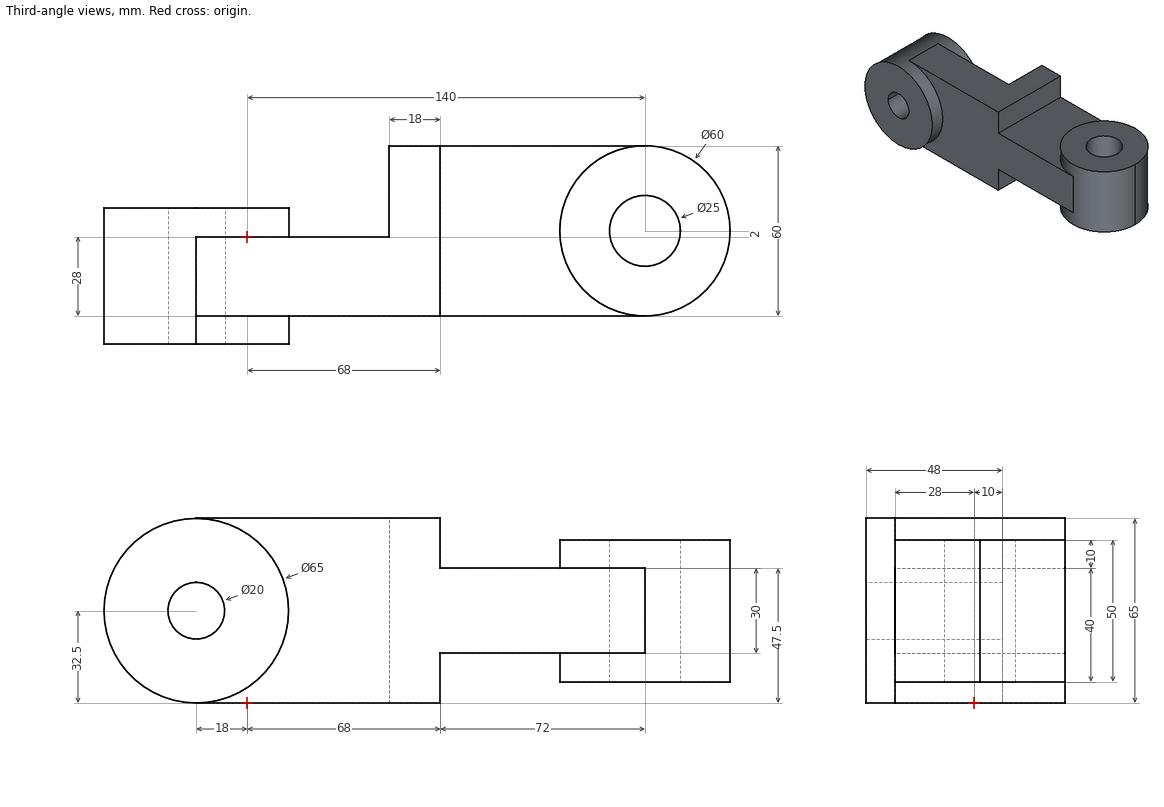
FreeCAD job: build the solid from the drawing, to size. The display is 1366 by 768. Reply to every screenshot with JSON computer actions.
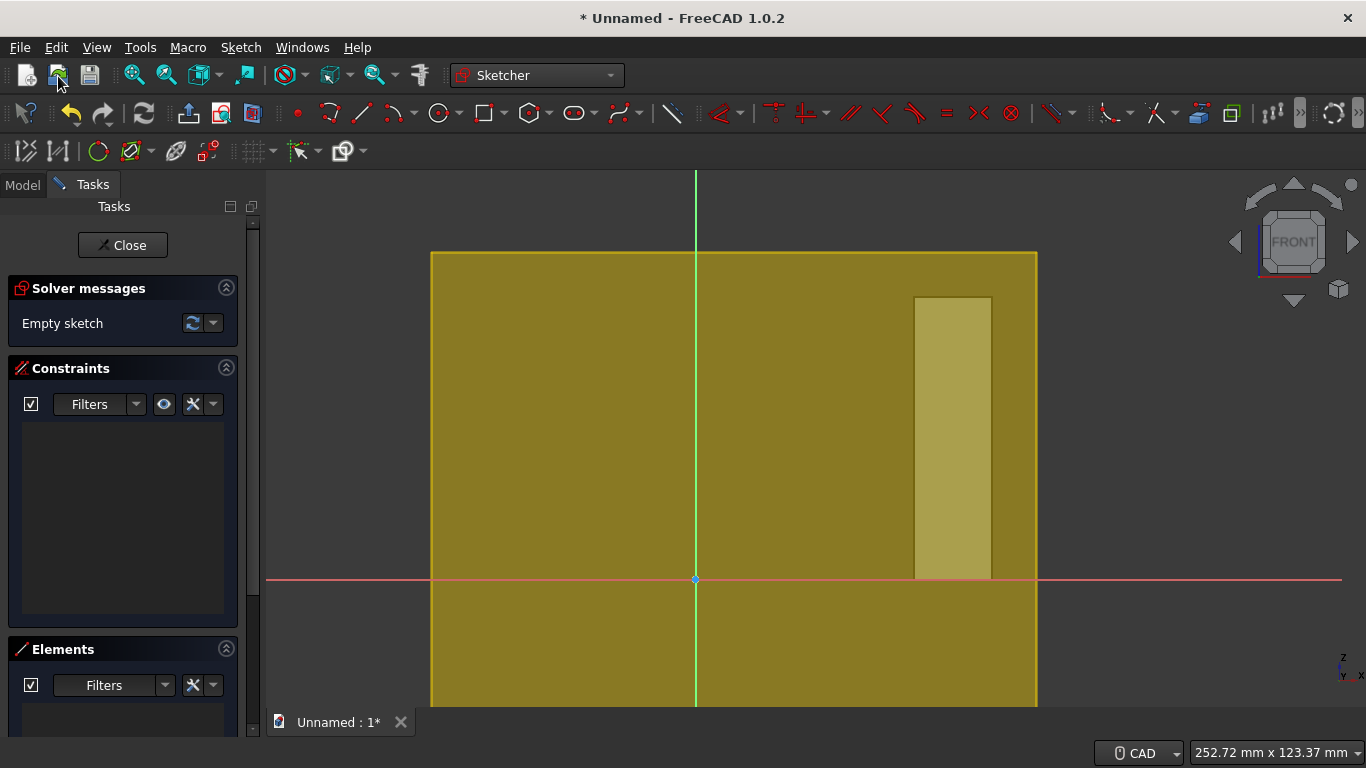
{"action": "key", "text": "g c"}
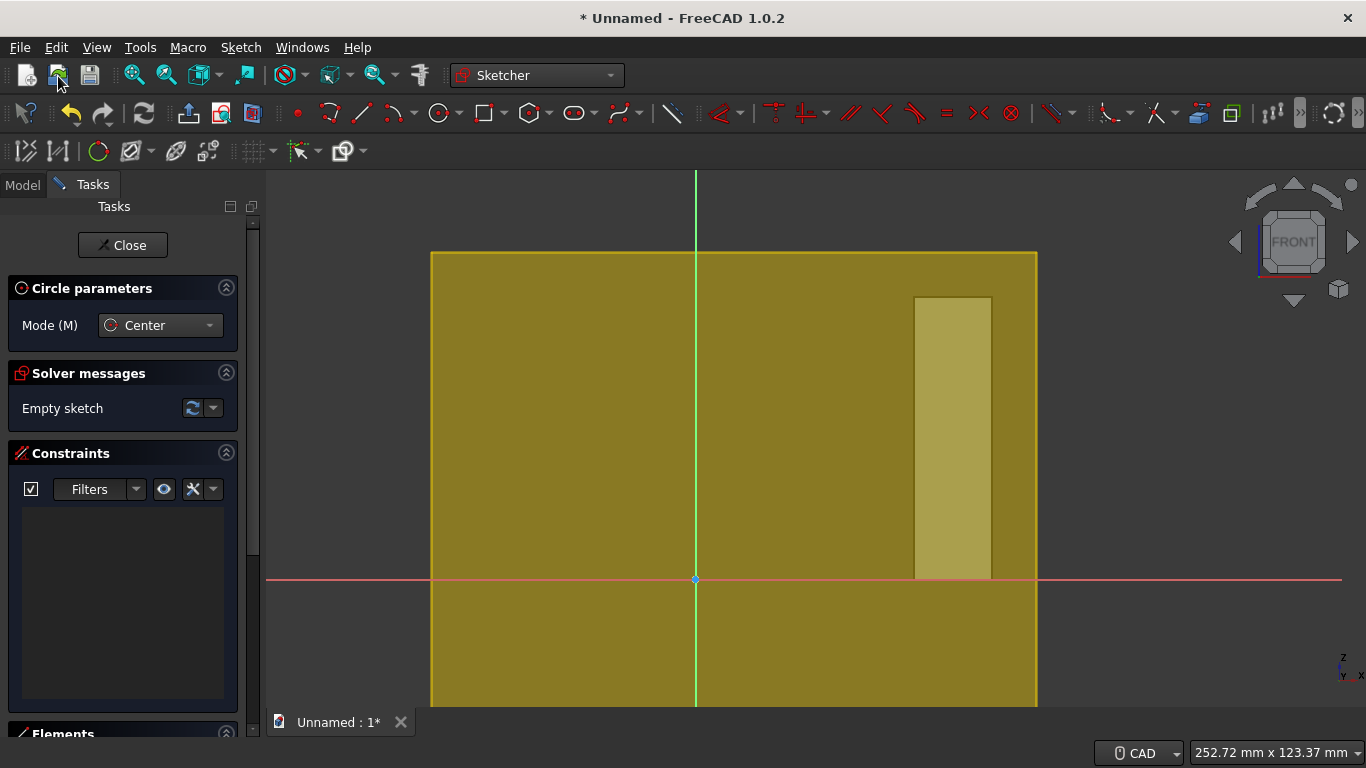
{"action": "left_click", "coordinate": [618, 439]}
{"action": "left_click", "coordinate": [718, 338]}
{"action": "key", "text": "Escape"}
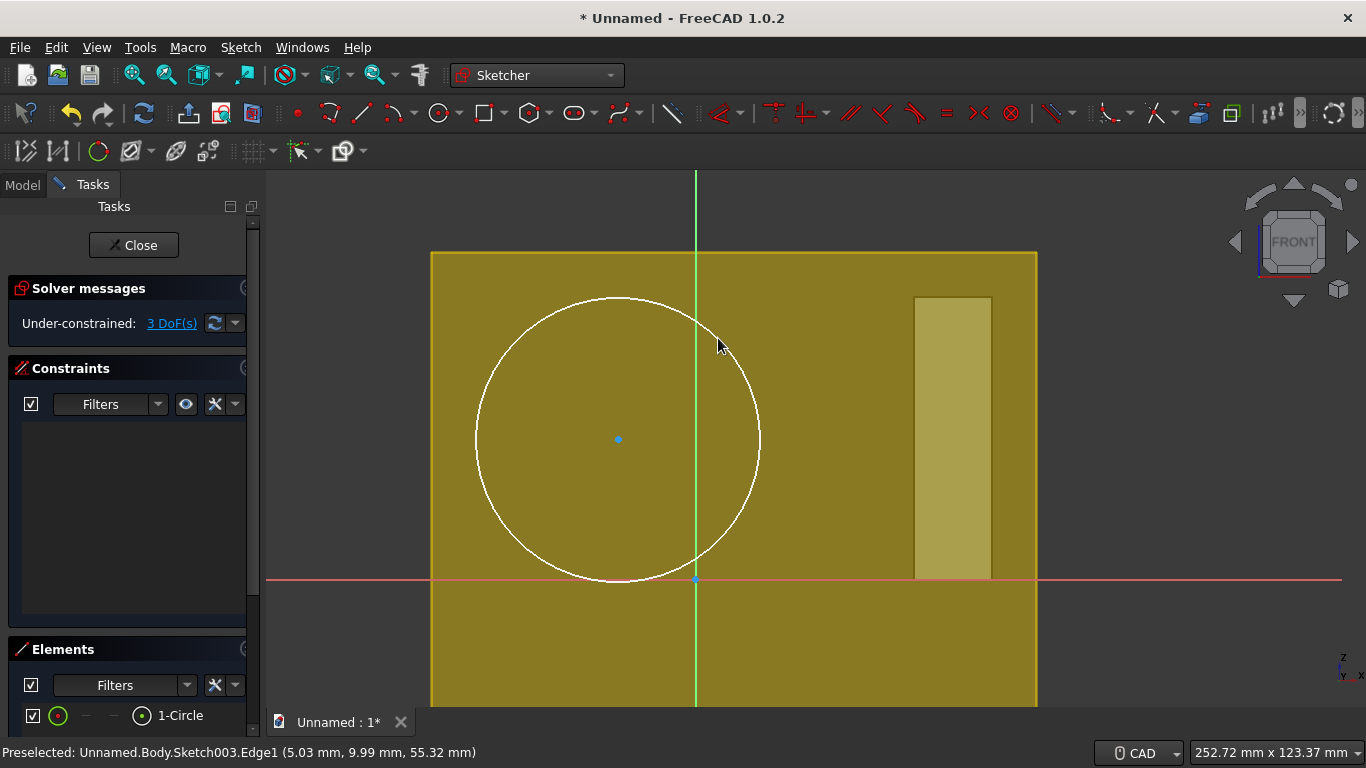
{"action": "key", "text": "d"}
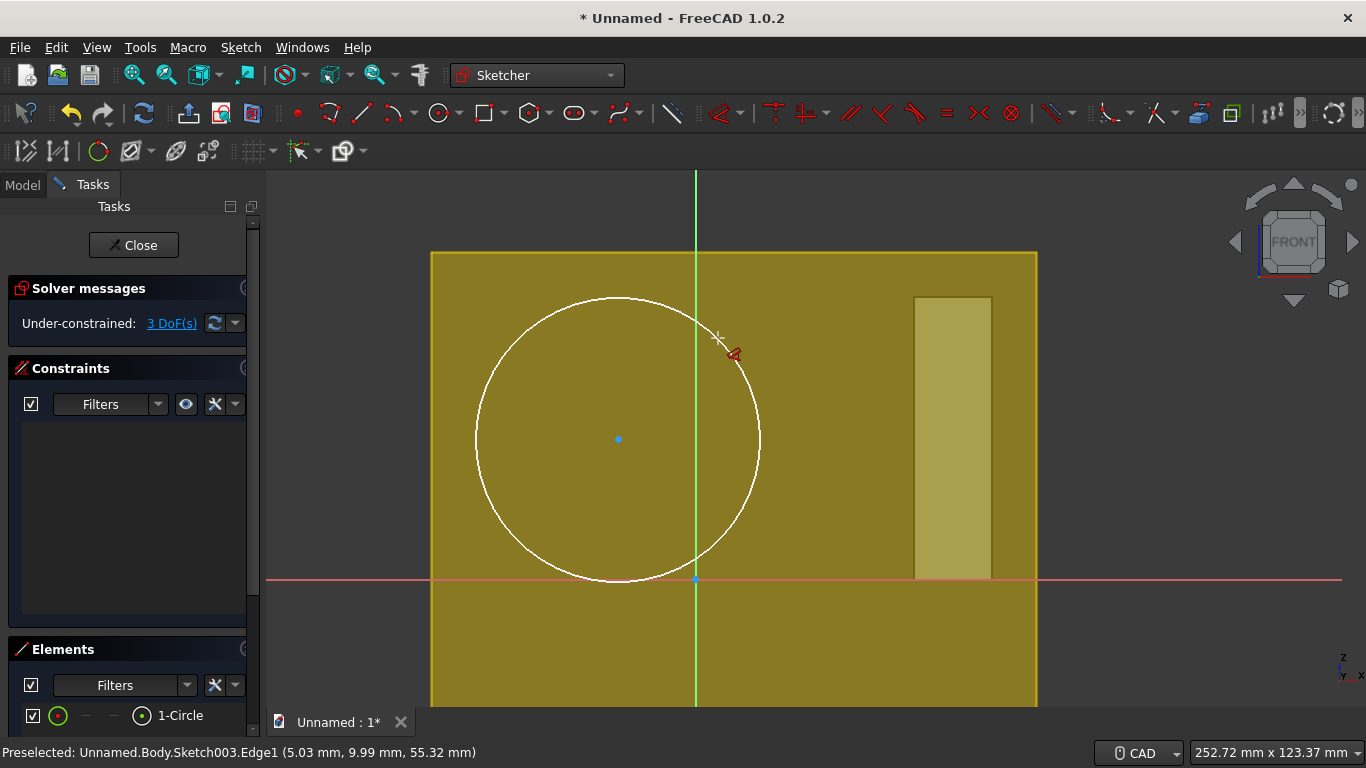
{"action": "left_click", "coordinate": [718, 339]}
{"action": "left_click", "coordinate": [741, 316]}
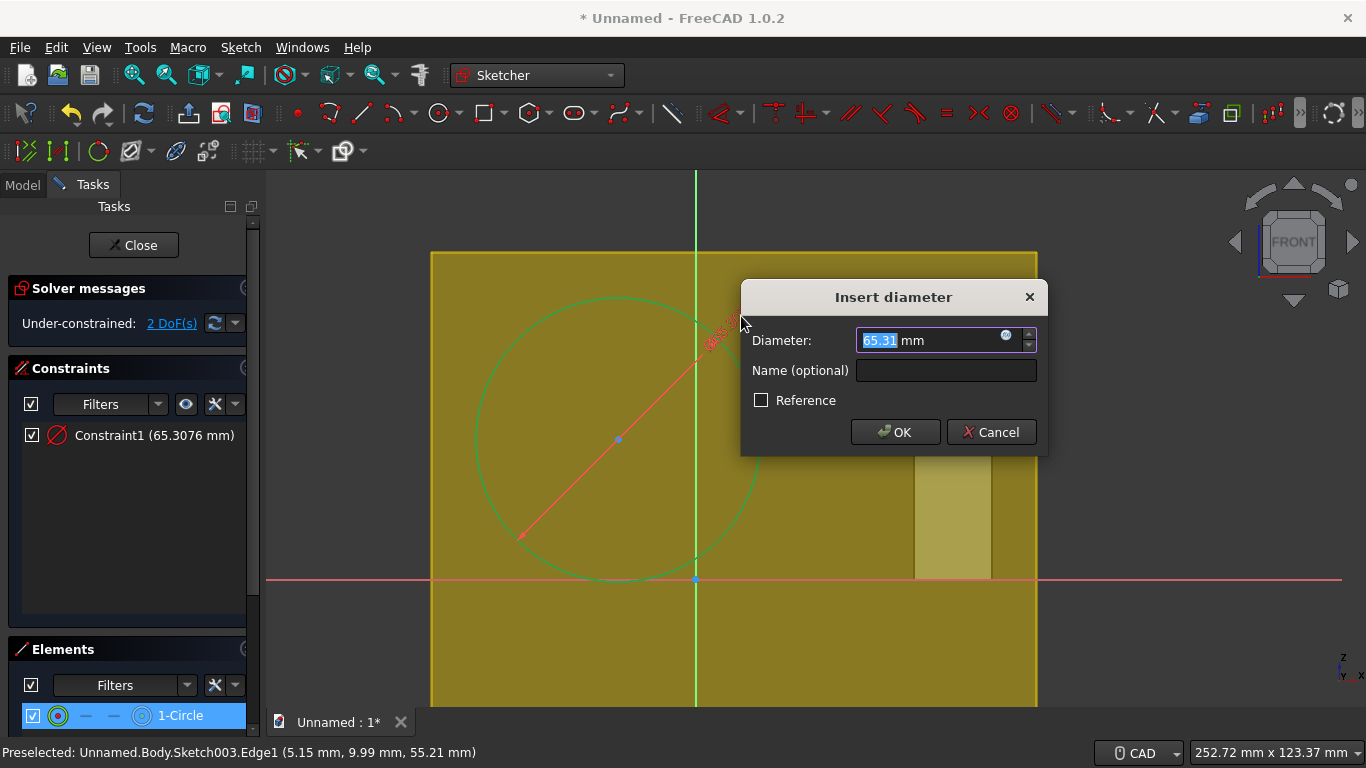
{"action": "type", "text": "65"}
{"action": "key", "text": "Return"}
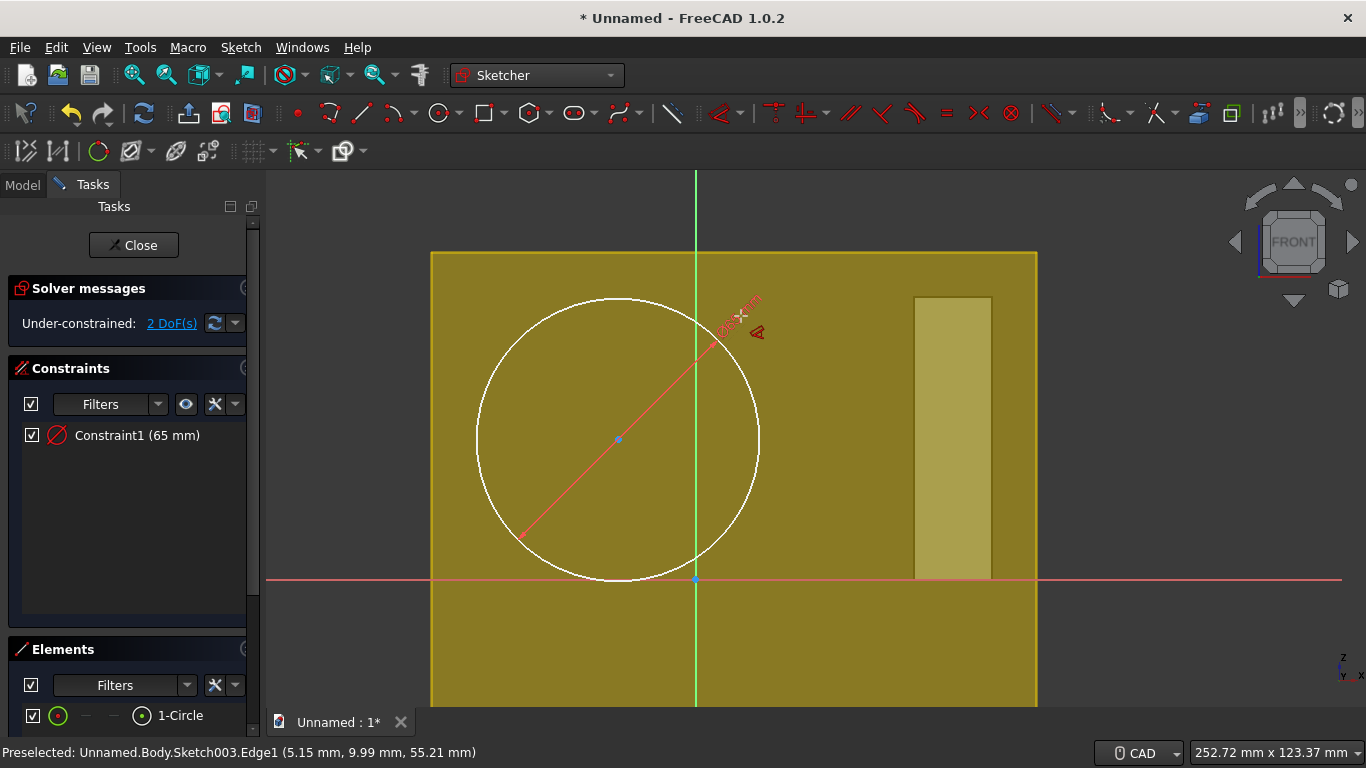
{"action": "left_click", "coordinate": [618, 440]}
{"action": "left_click", "coordinate": [657, 614]}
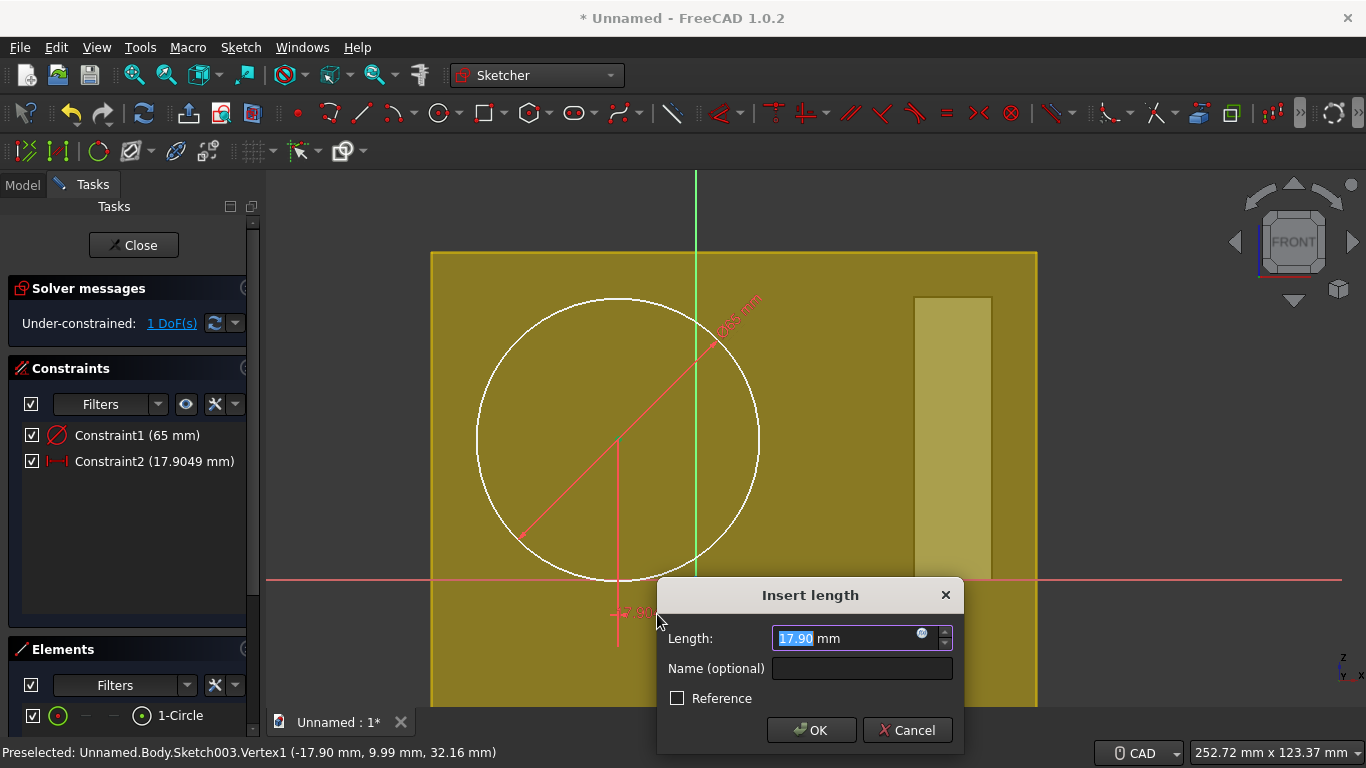
{"action": "type", "text": "18"}
{"action": "key", "text": "Return"}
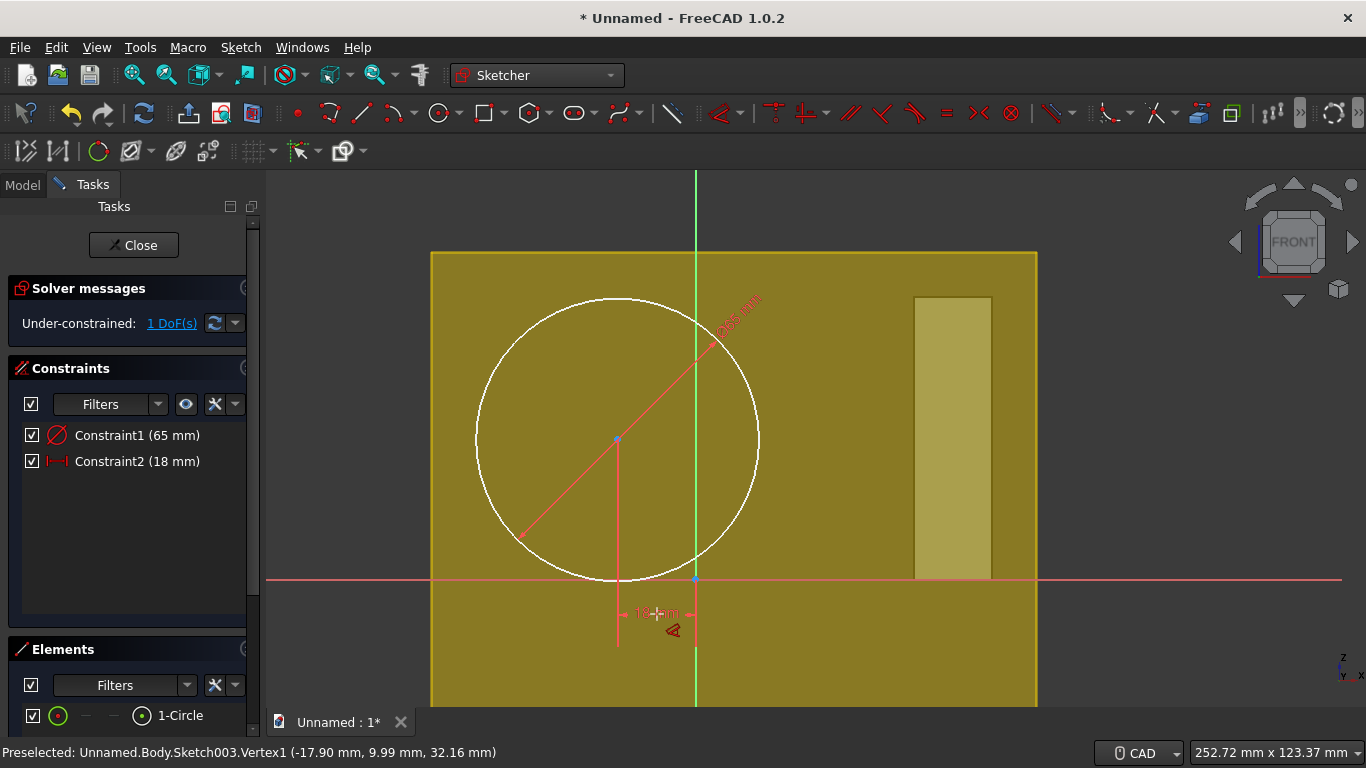
{"action": "left_click", "coordinate": [618, 440]}
{"action": "left_click", "coordinate": [730, 478]}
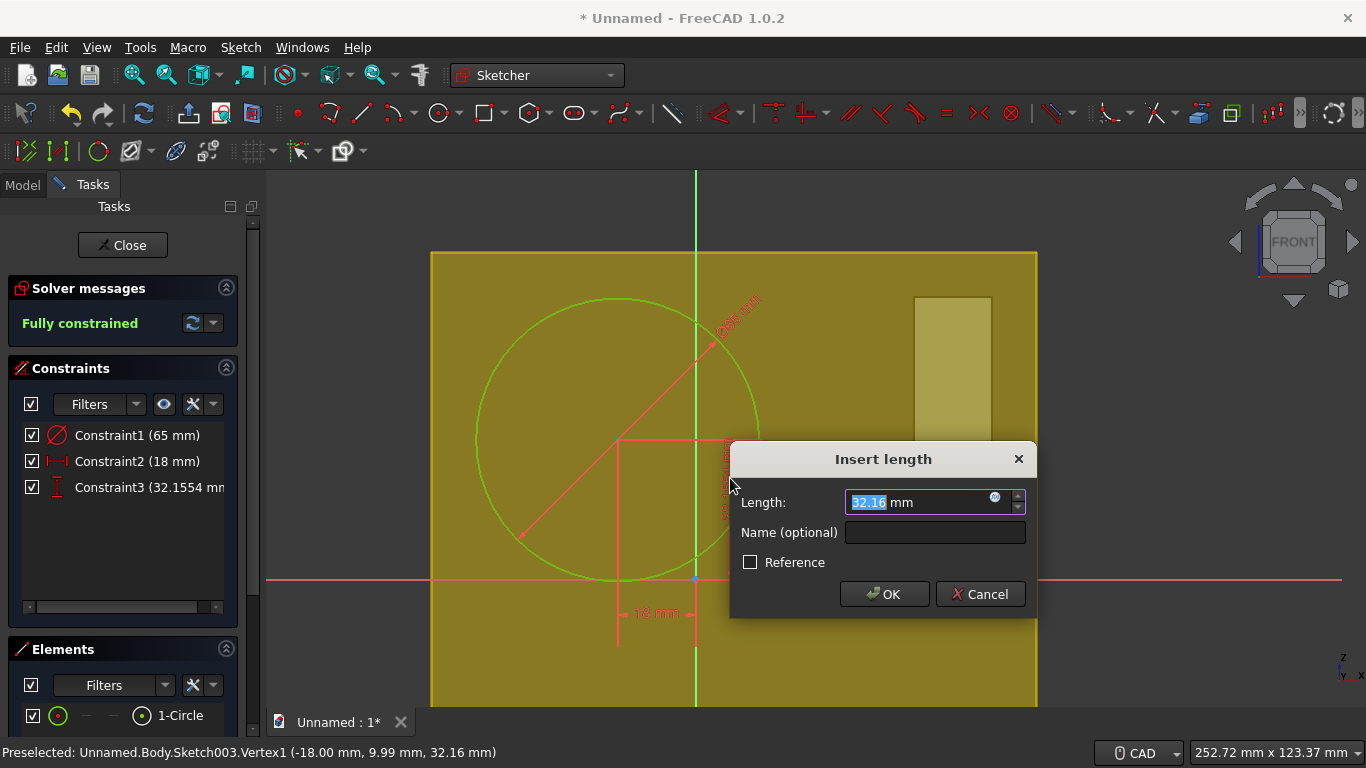
{"action": "type", "text": "32.5"}
{"action": "key", "text": "Return"}
{"action": "key", "text": "Escape"}